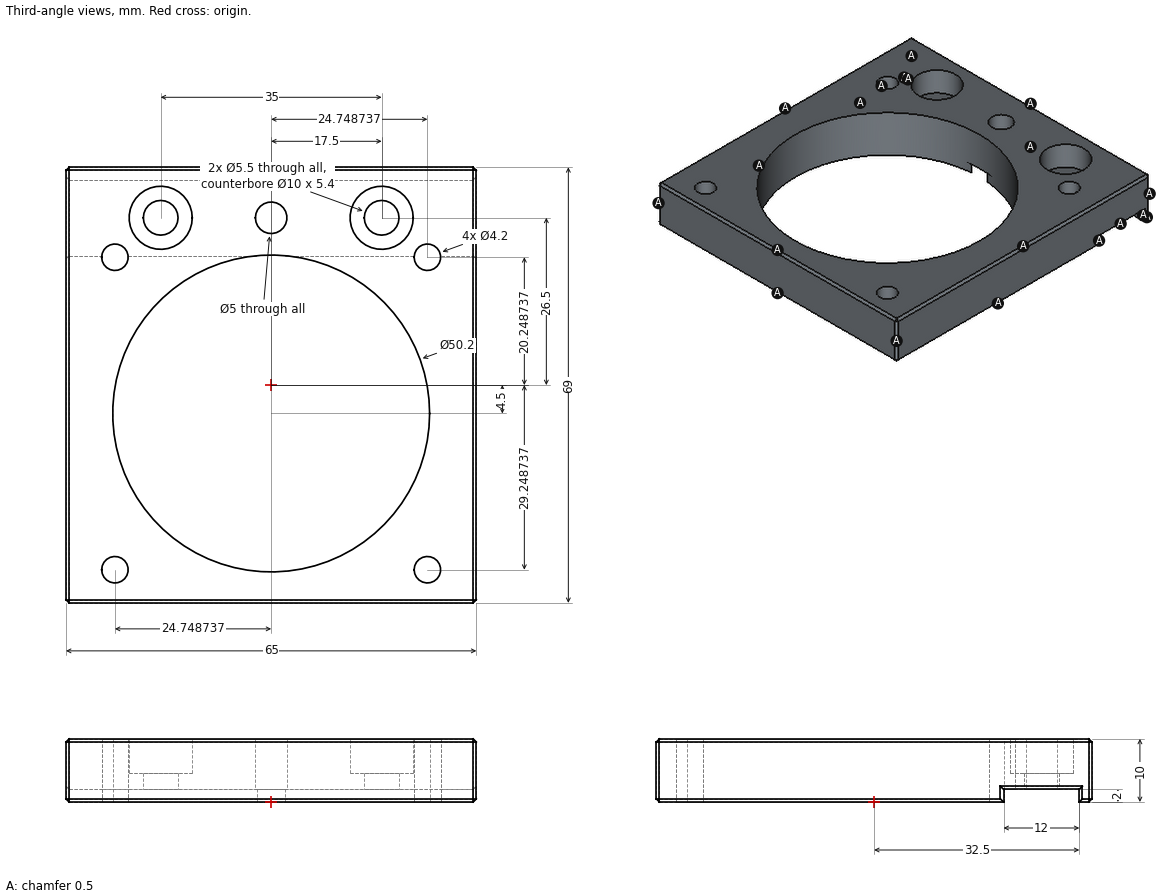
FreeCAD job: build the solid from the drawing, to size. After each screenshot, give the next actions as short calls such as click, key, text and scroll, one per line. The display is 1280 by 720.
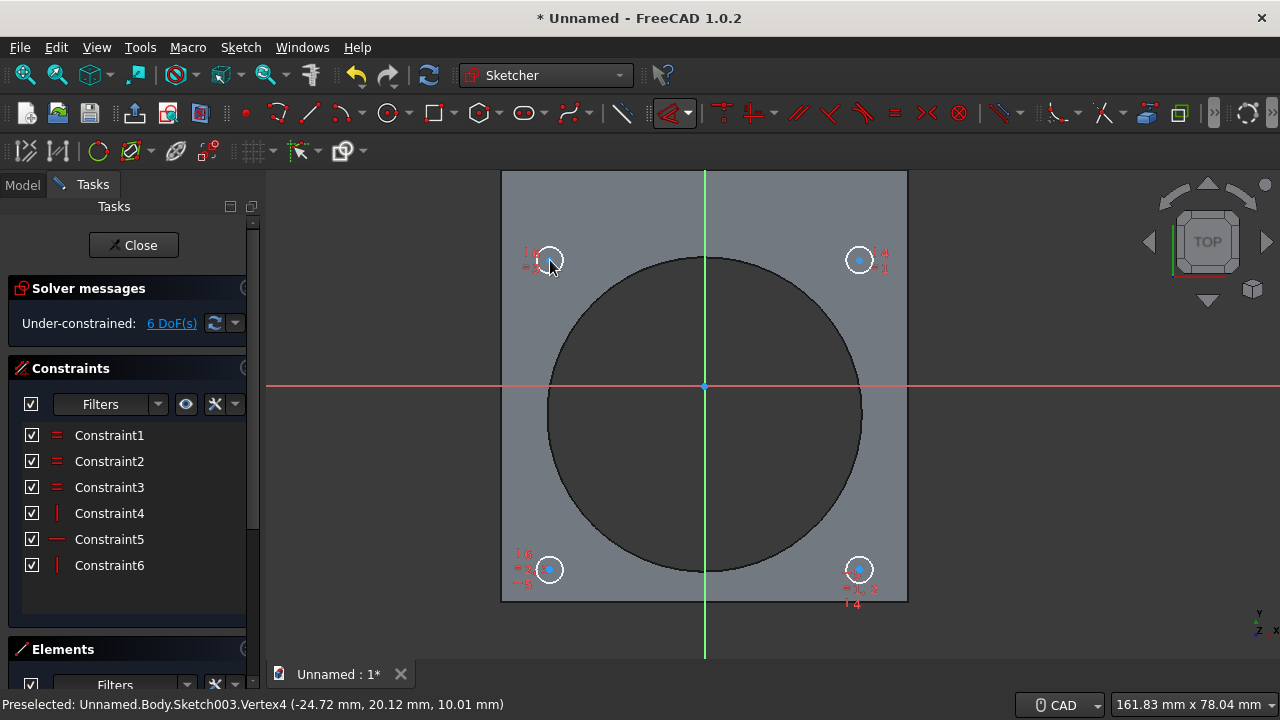
click(860, 260)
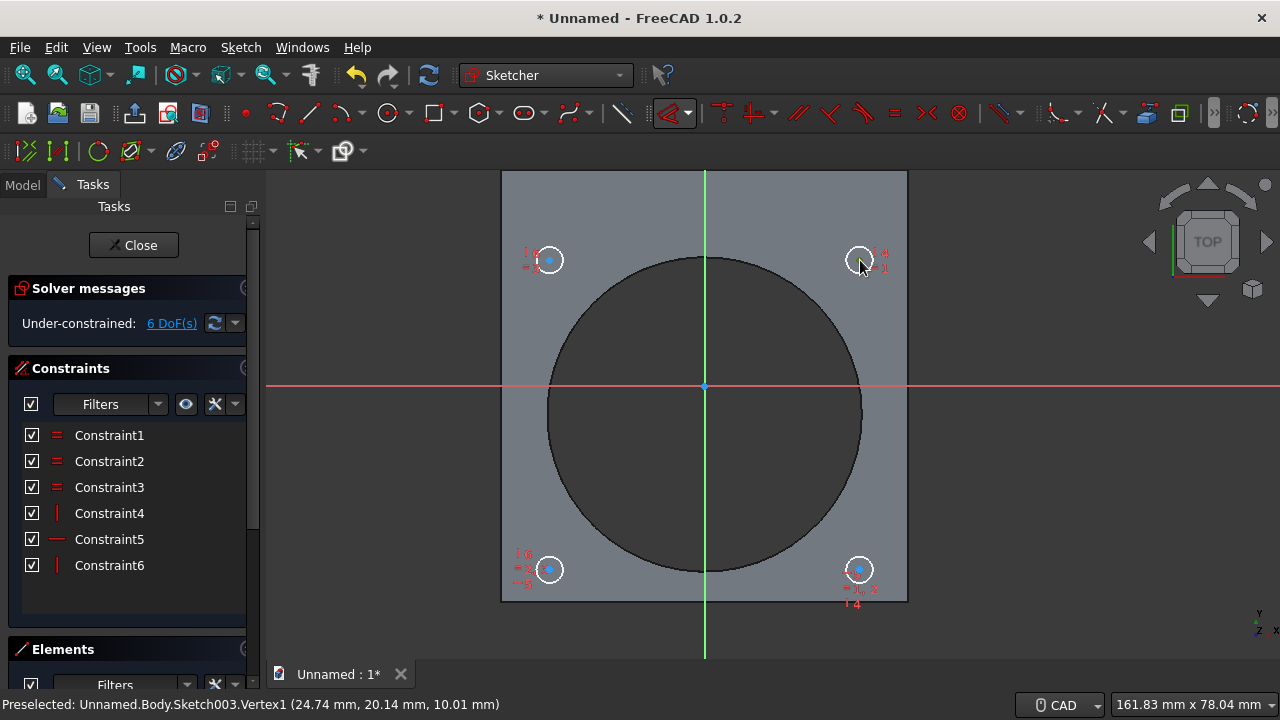
click(550, 260)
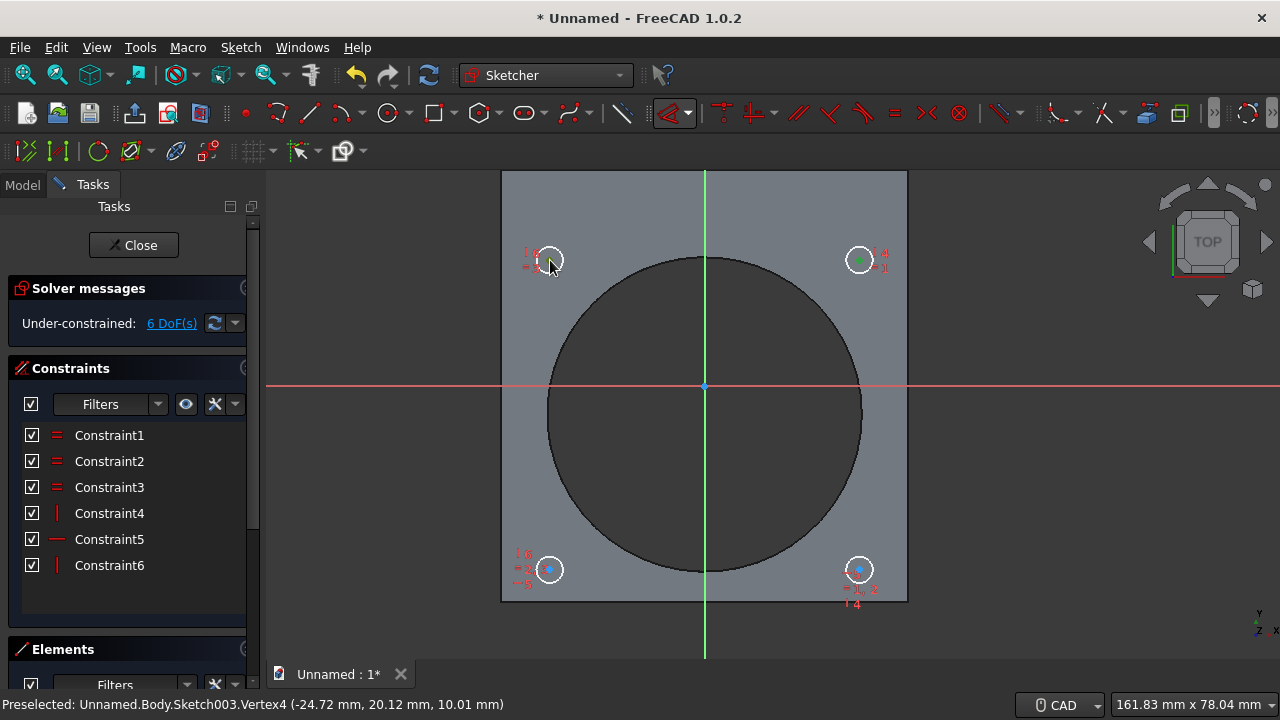
key(h)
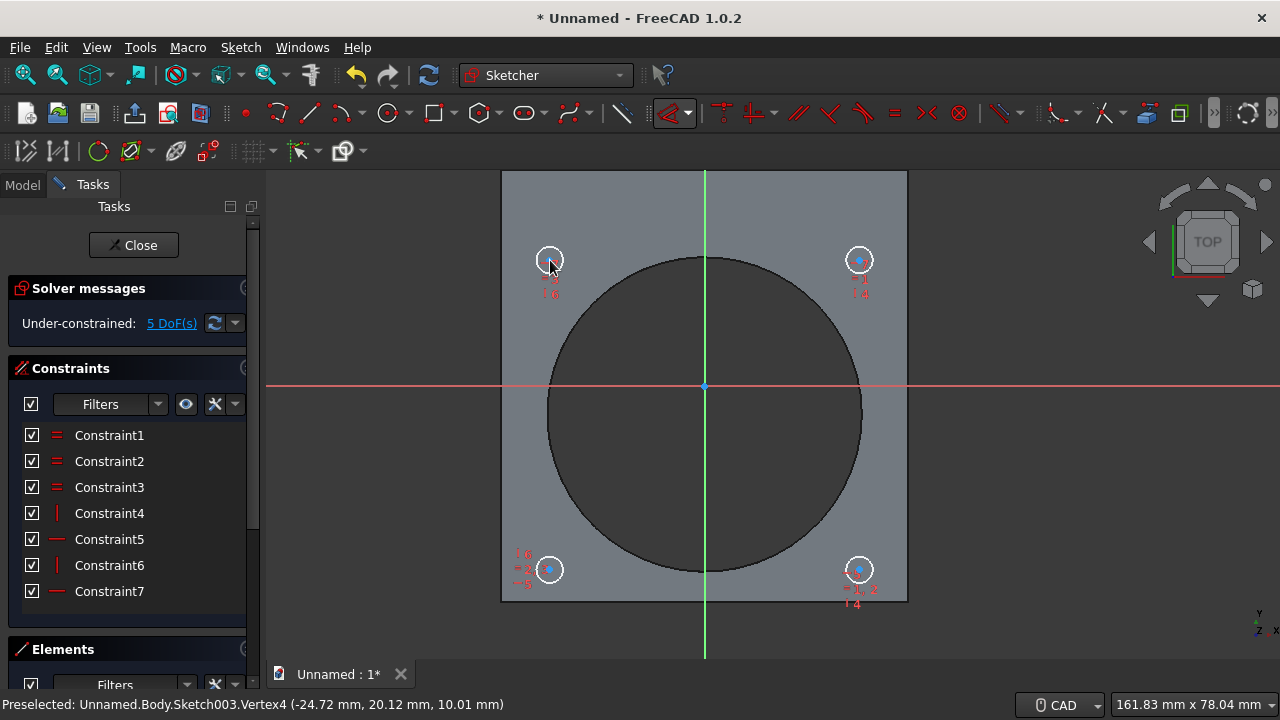
scroll(869, 251, up, 3)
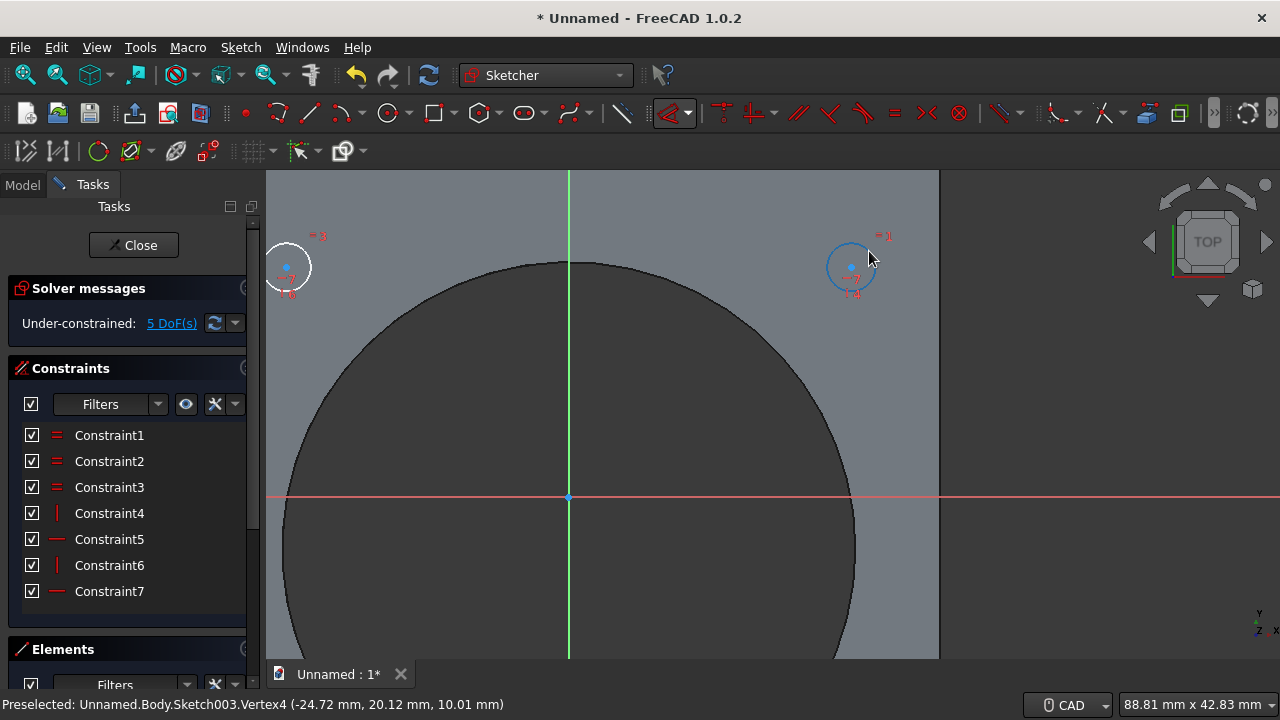
click(868, 250)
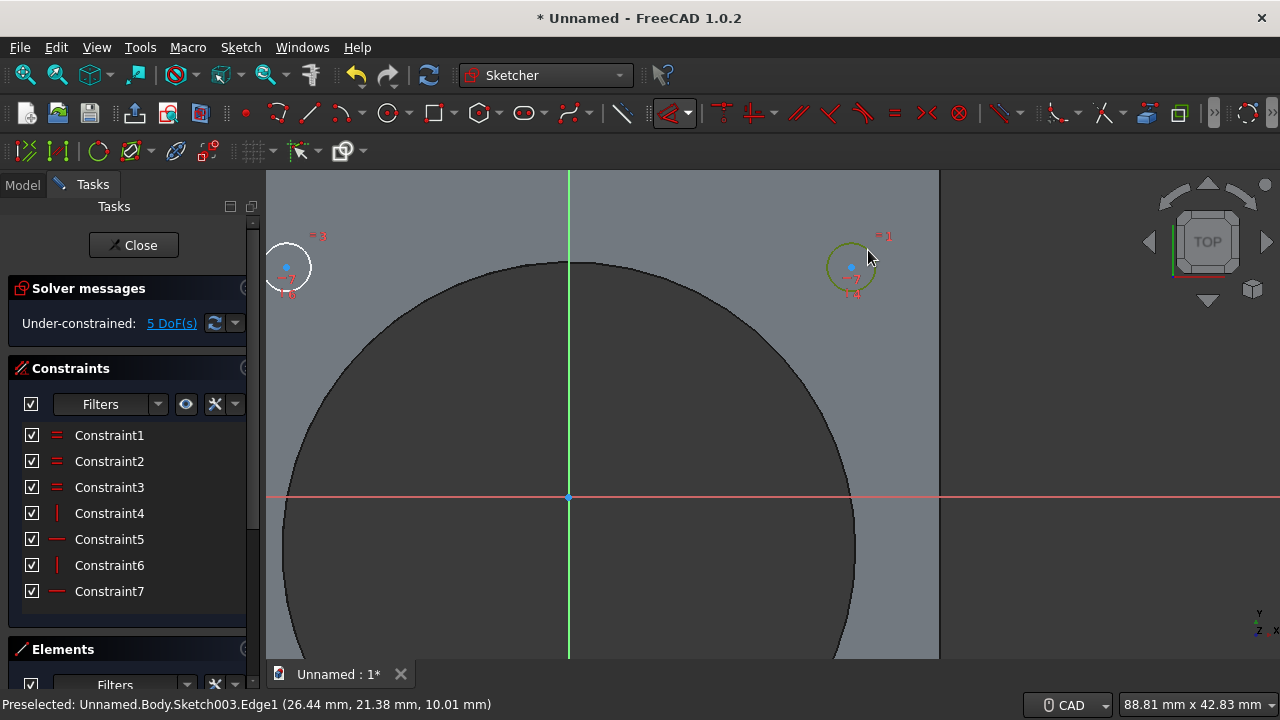
click(690, 114)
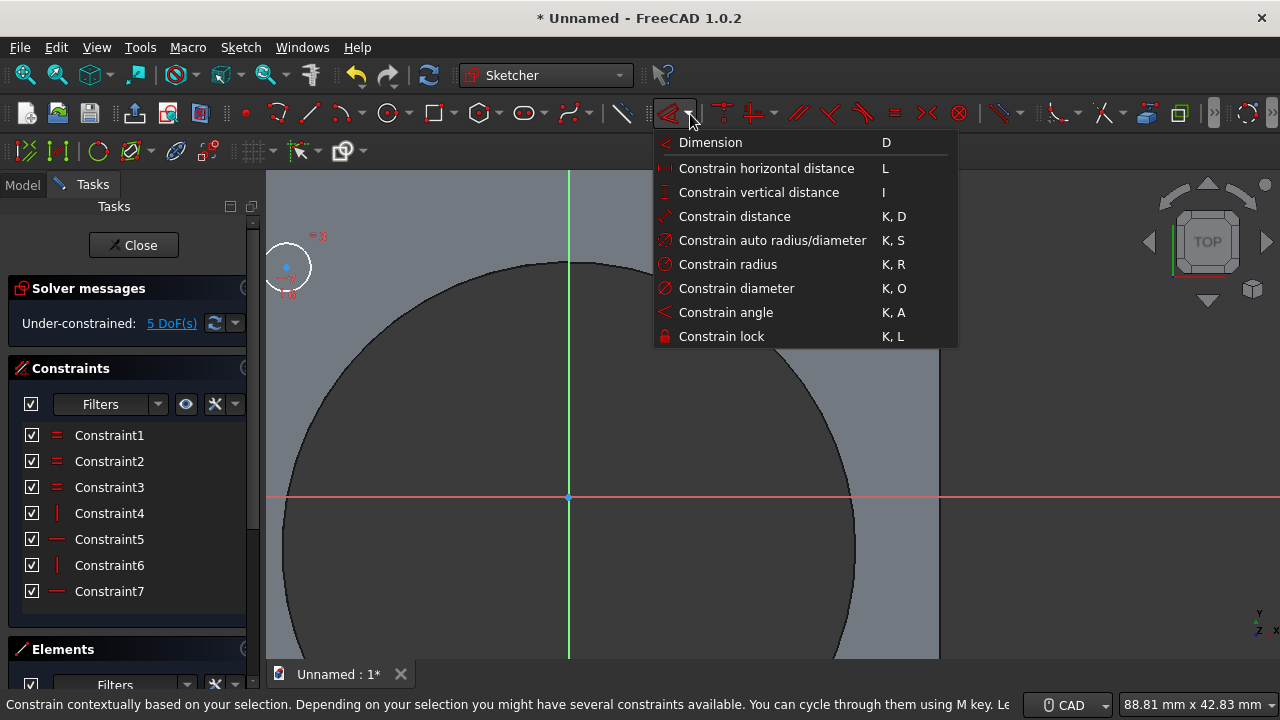
click(806, 288)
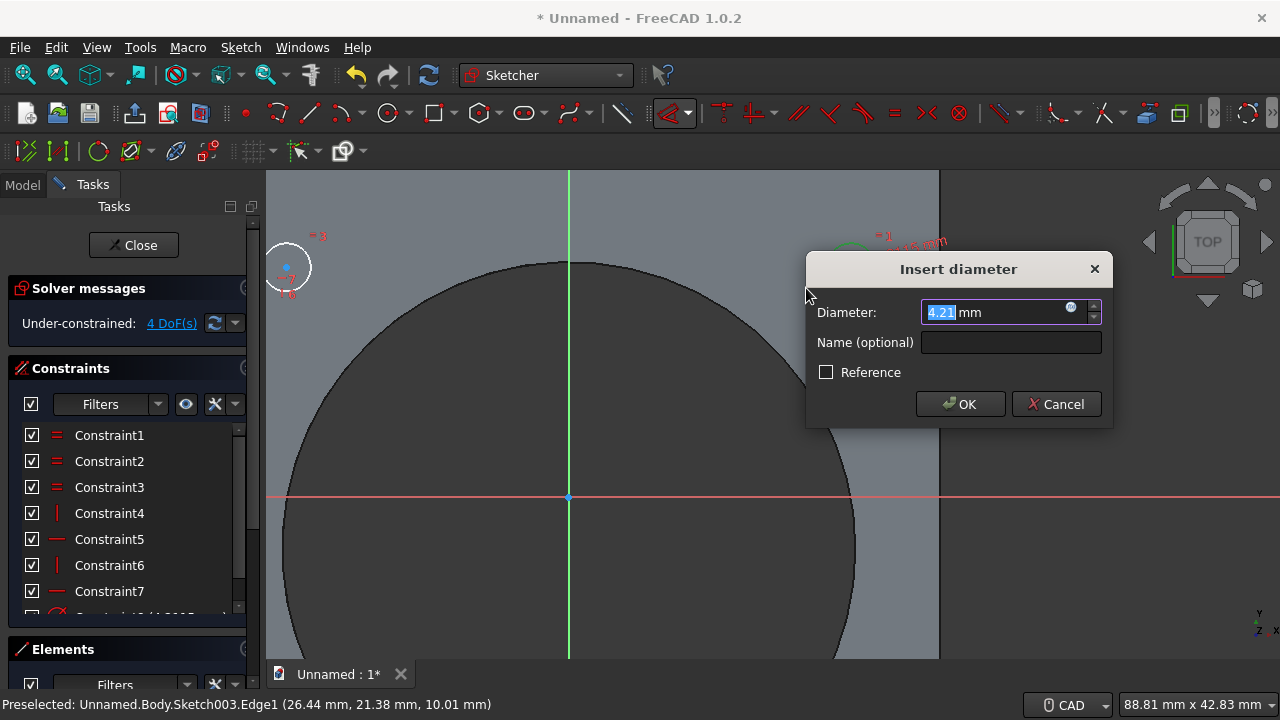
text(4.2)
key(Return)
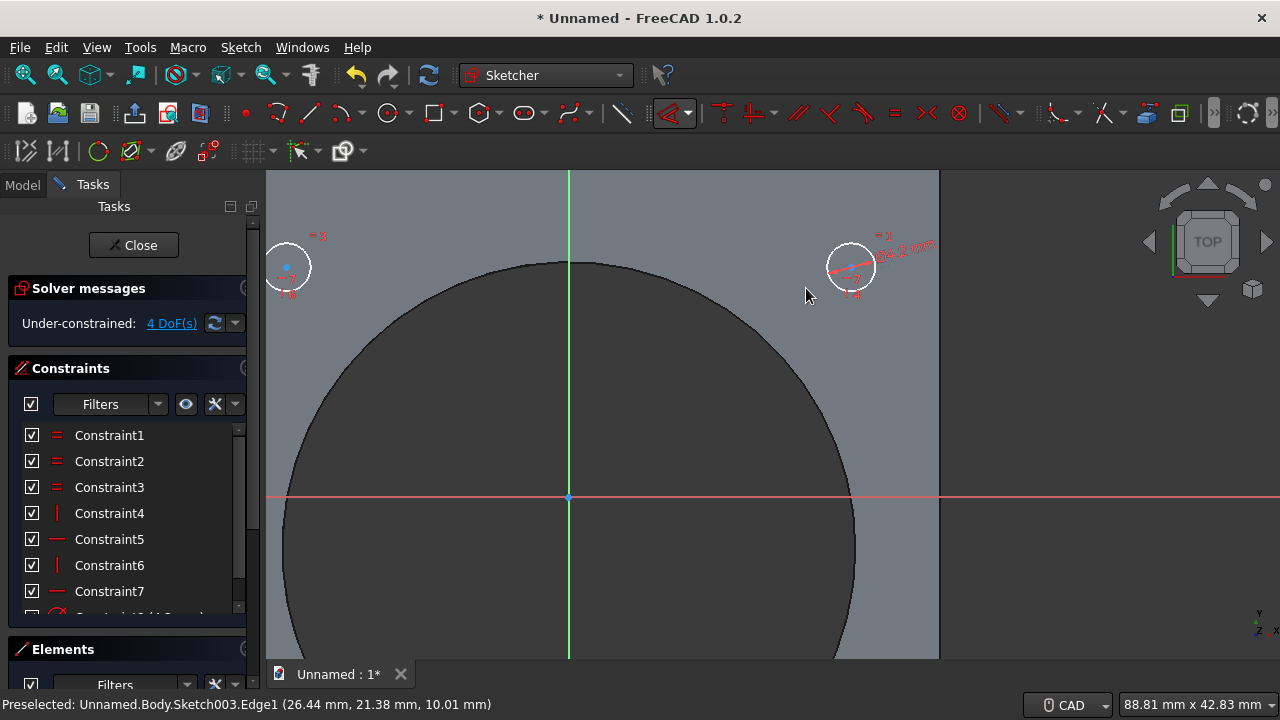
click(851, 267)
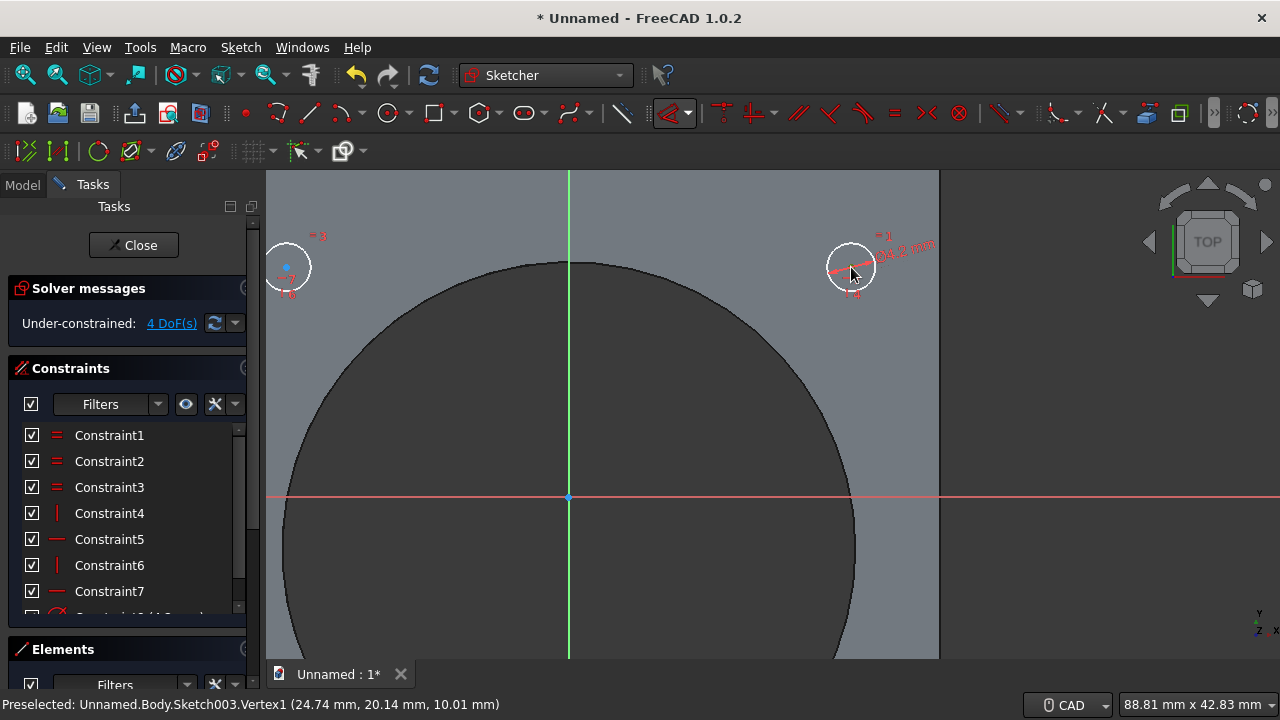
key(l)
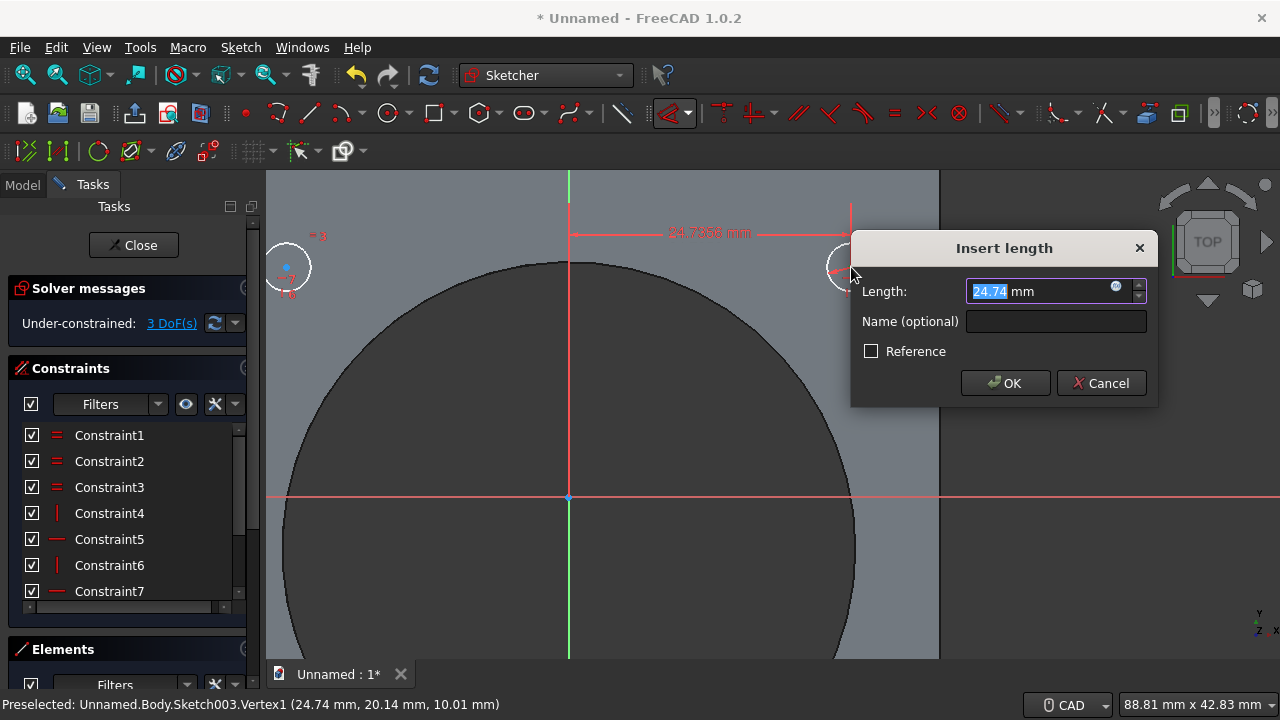
text(24.748737)
key(Return)